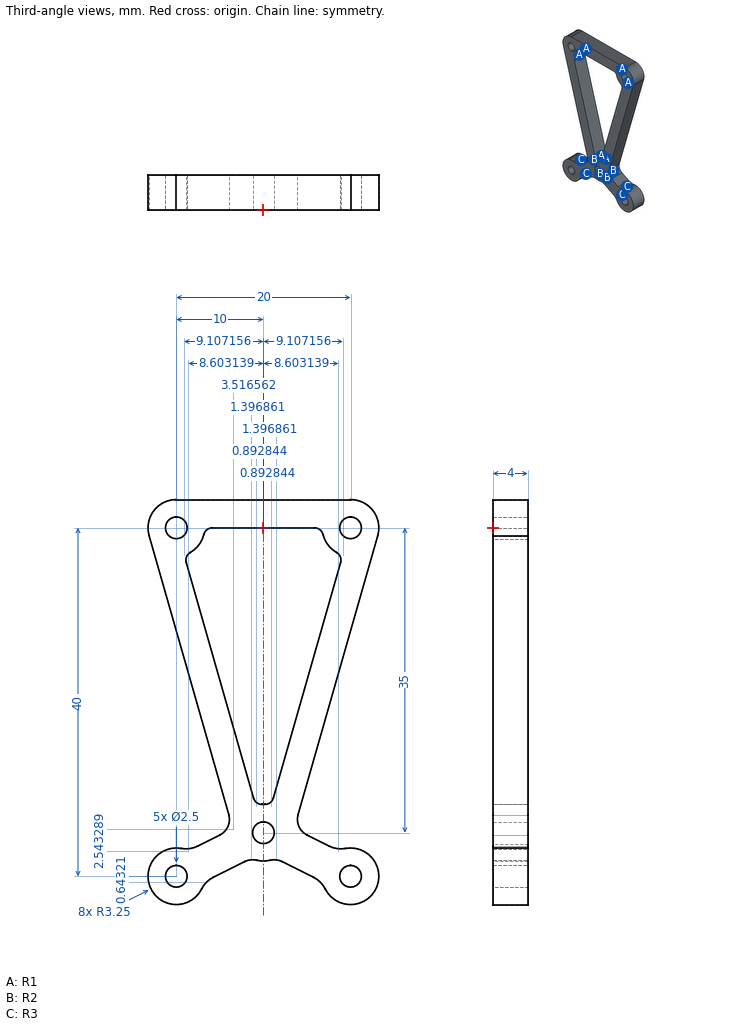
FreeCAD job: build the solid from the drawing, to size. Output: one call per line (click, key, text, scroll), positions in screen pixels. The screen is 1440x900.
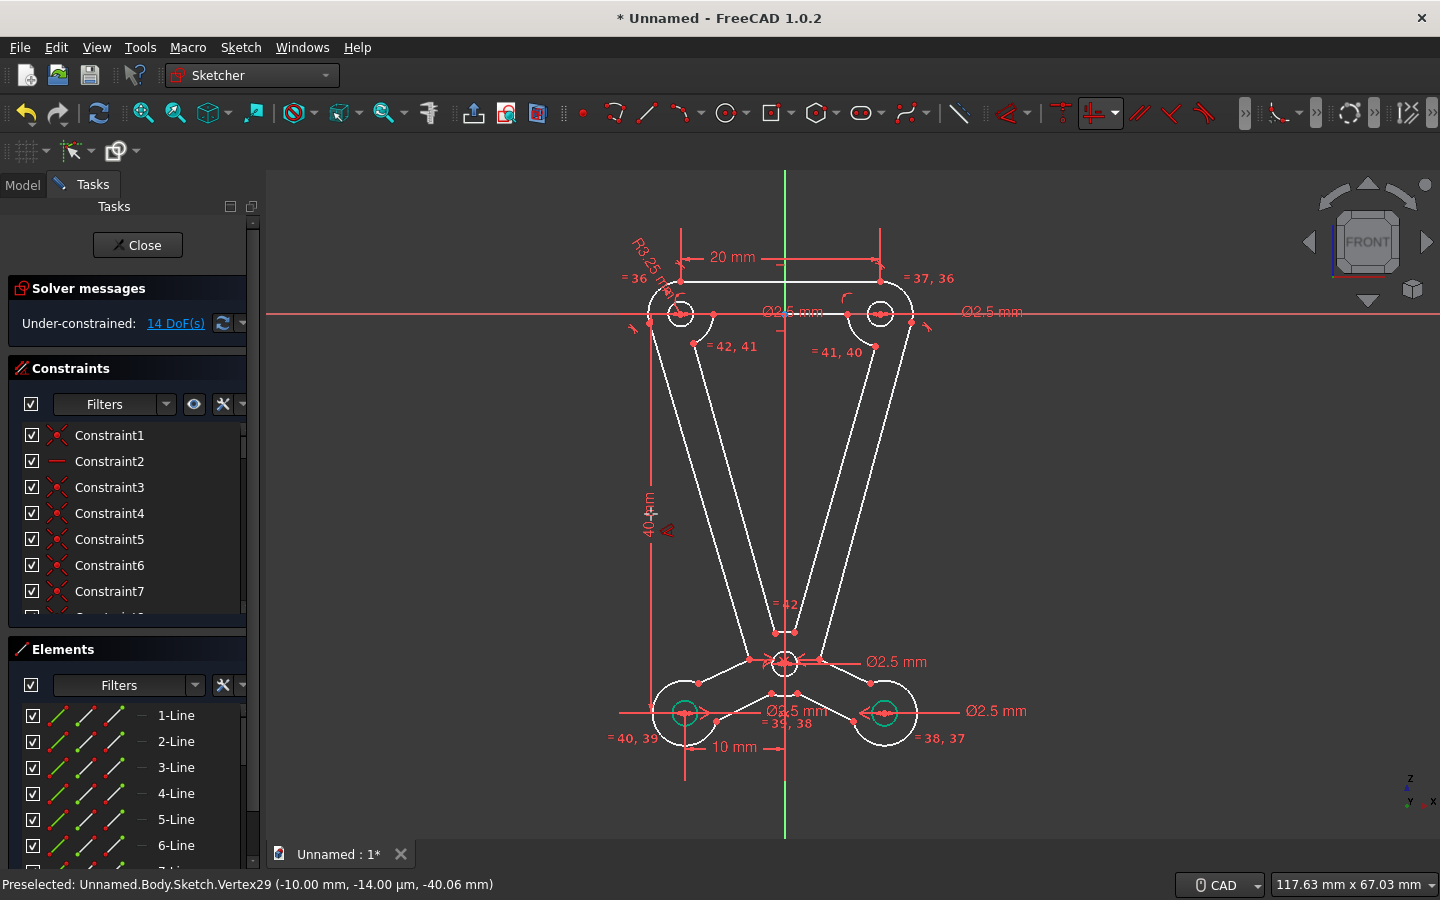
click(785, 664)
click(819, 489)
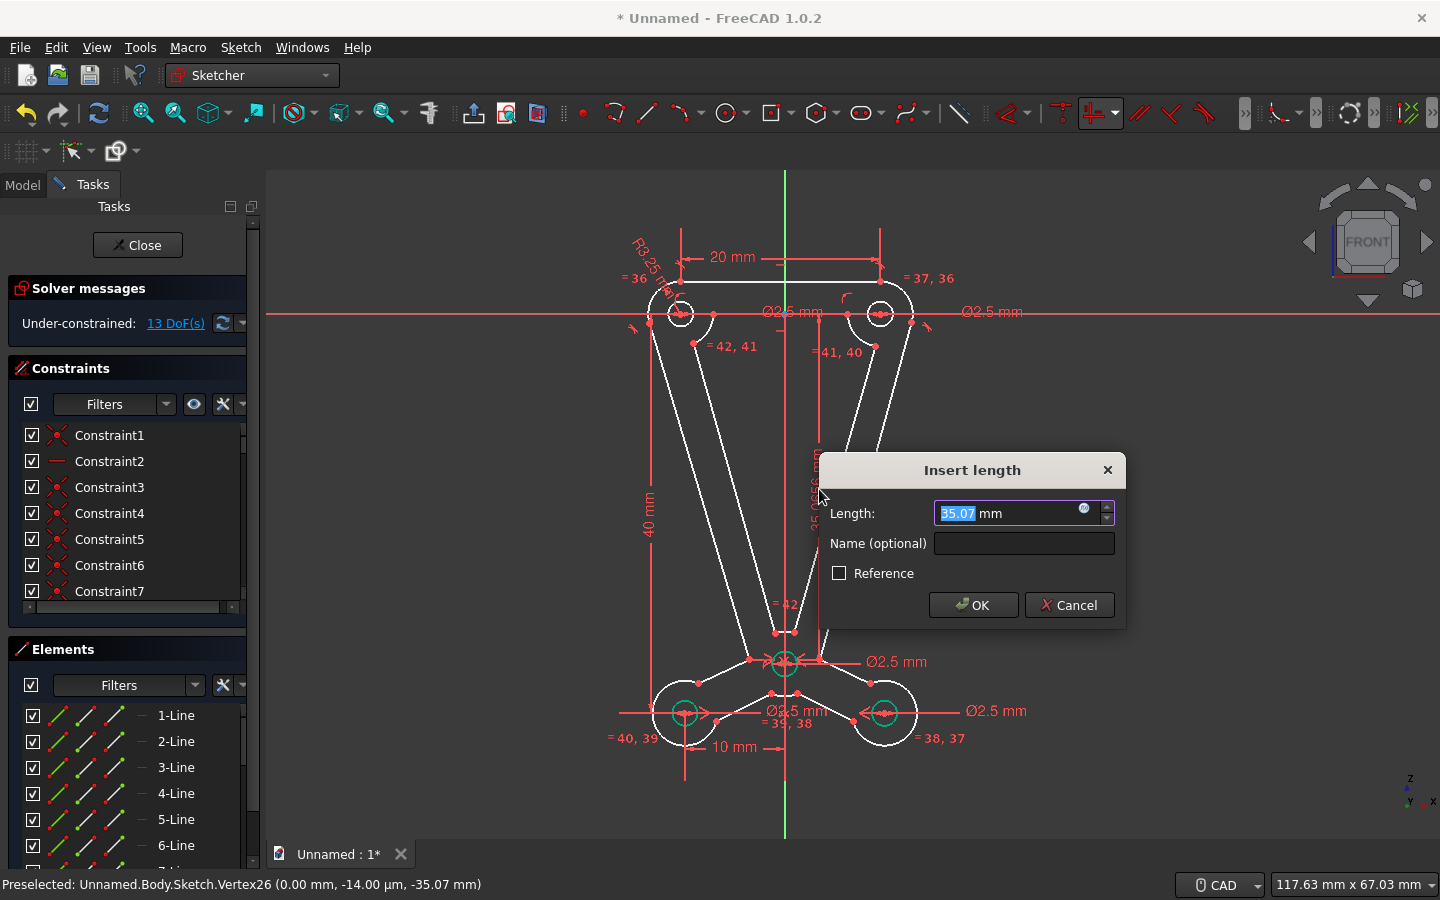
text(35)
key(Return)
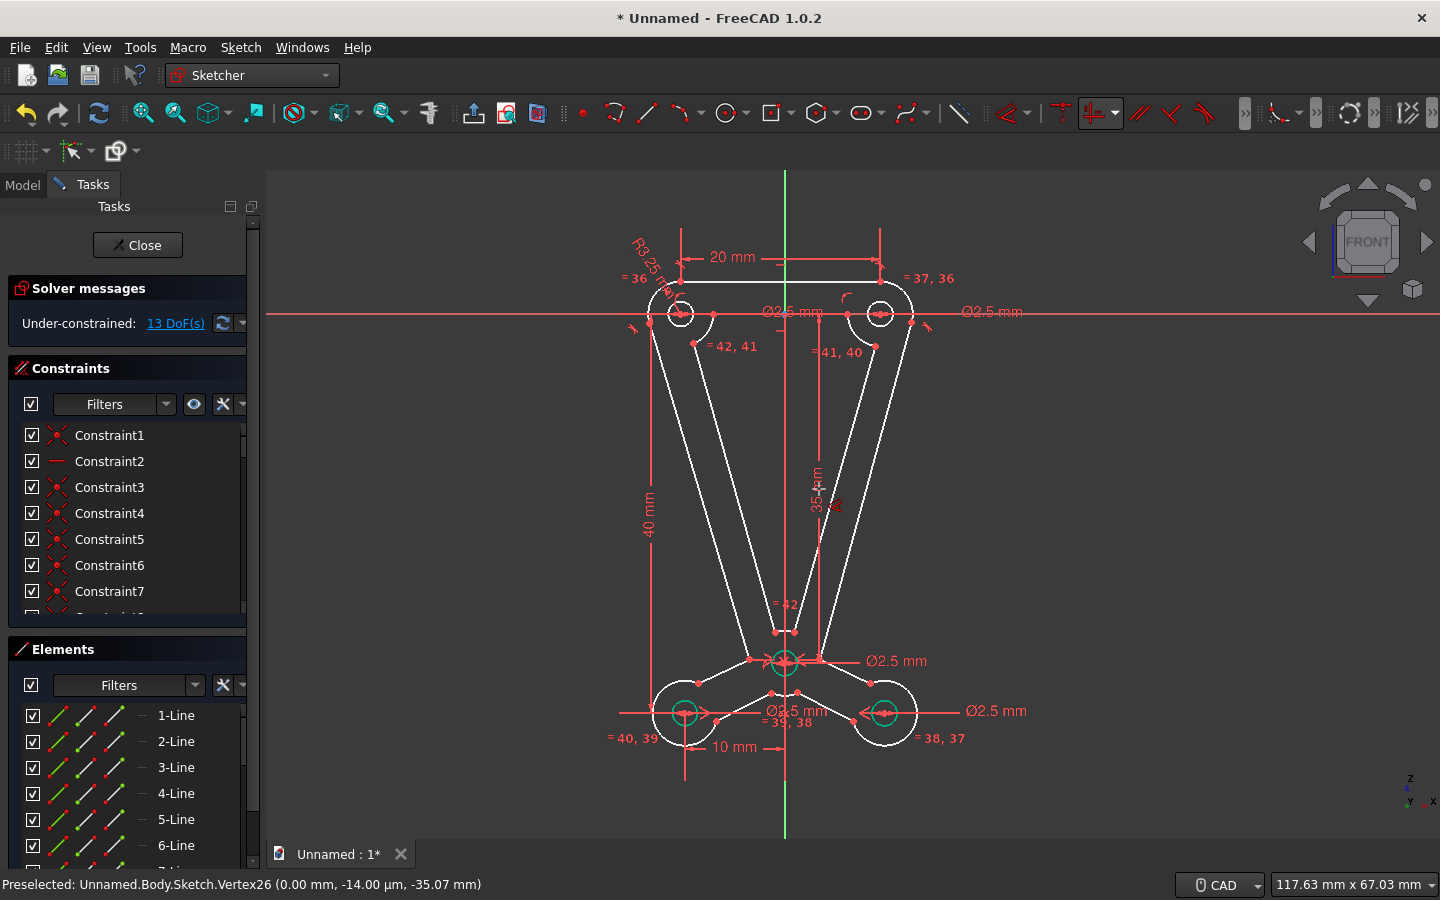
click(681, 314)
click(733, 348)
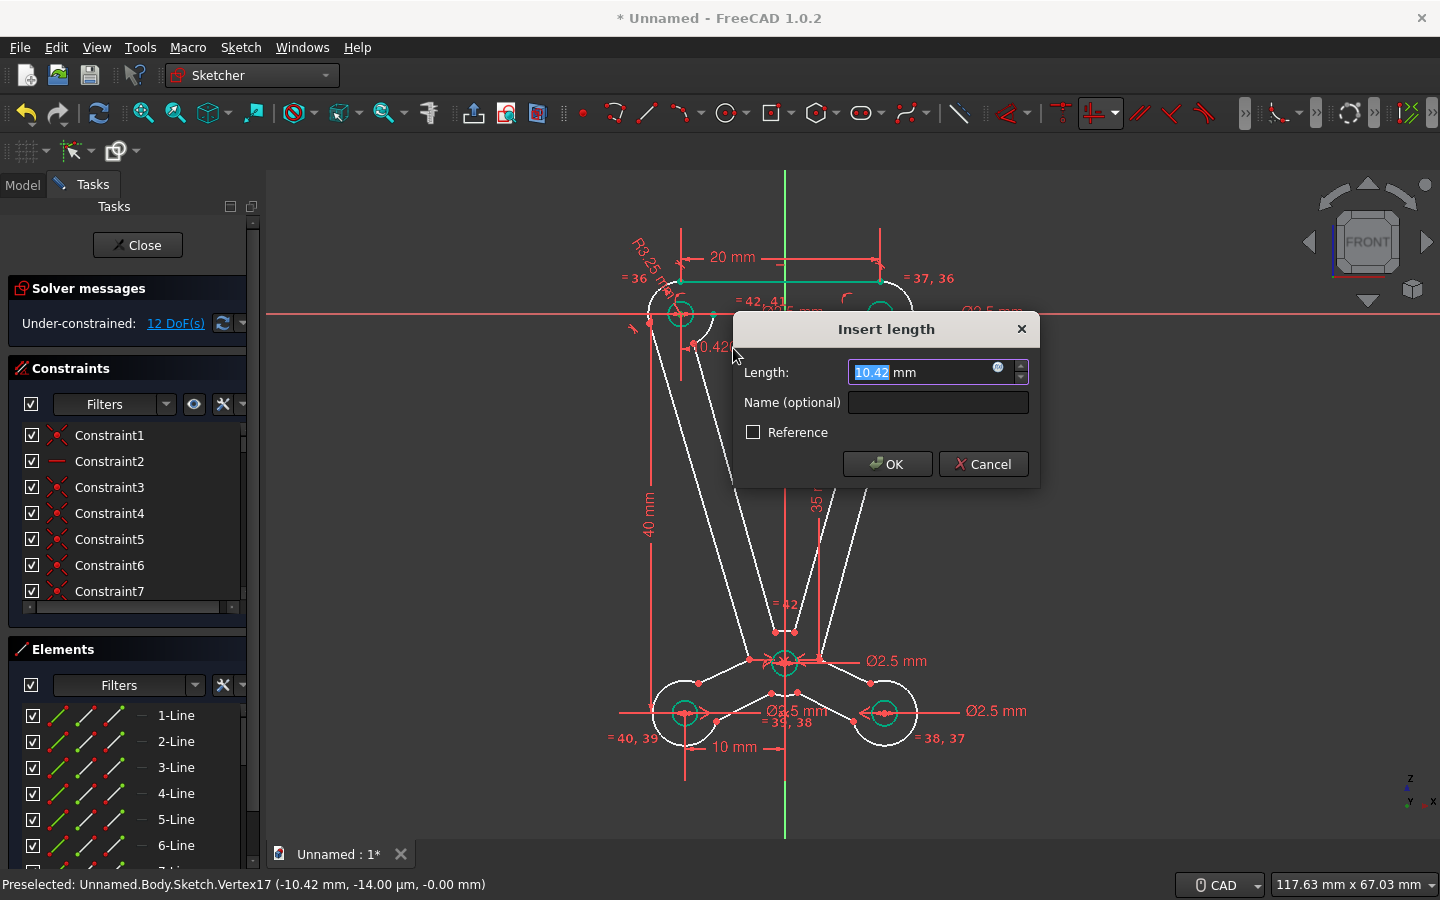
text(10)
key(Return)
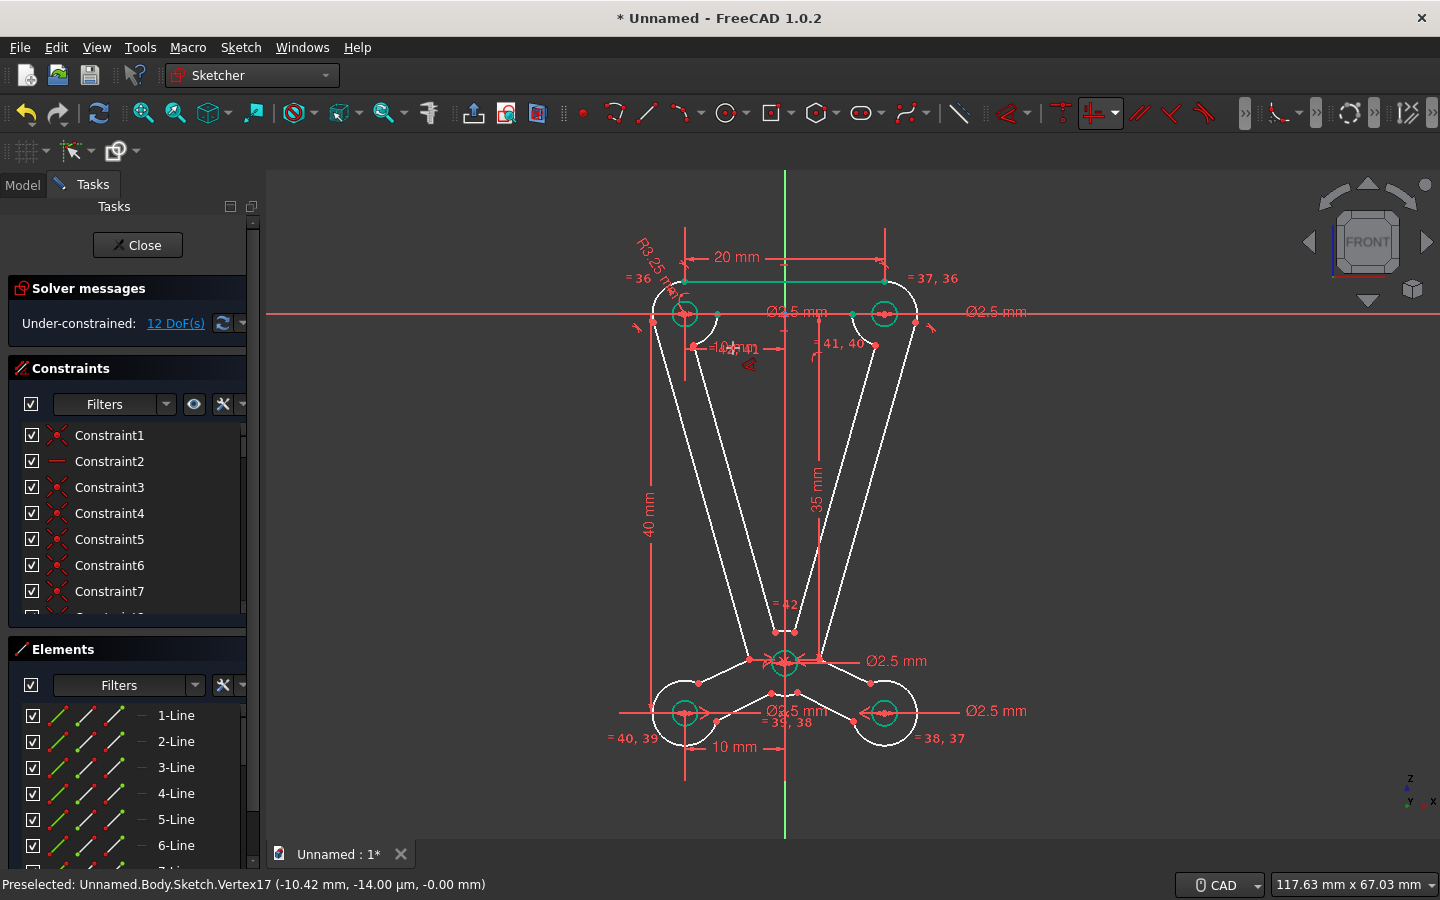
scroll(716, 721, up, 10)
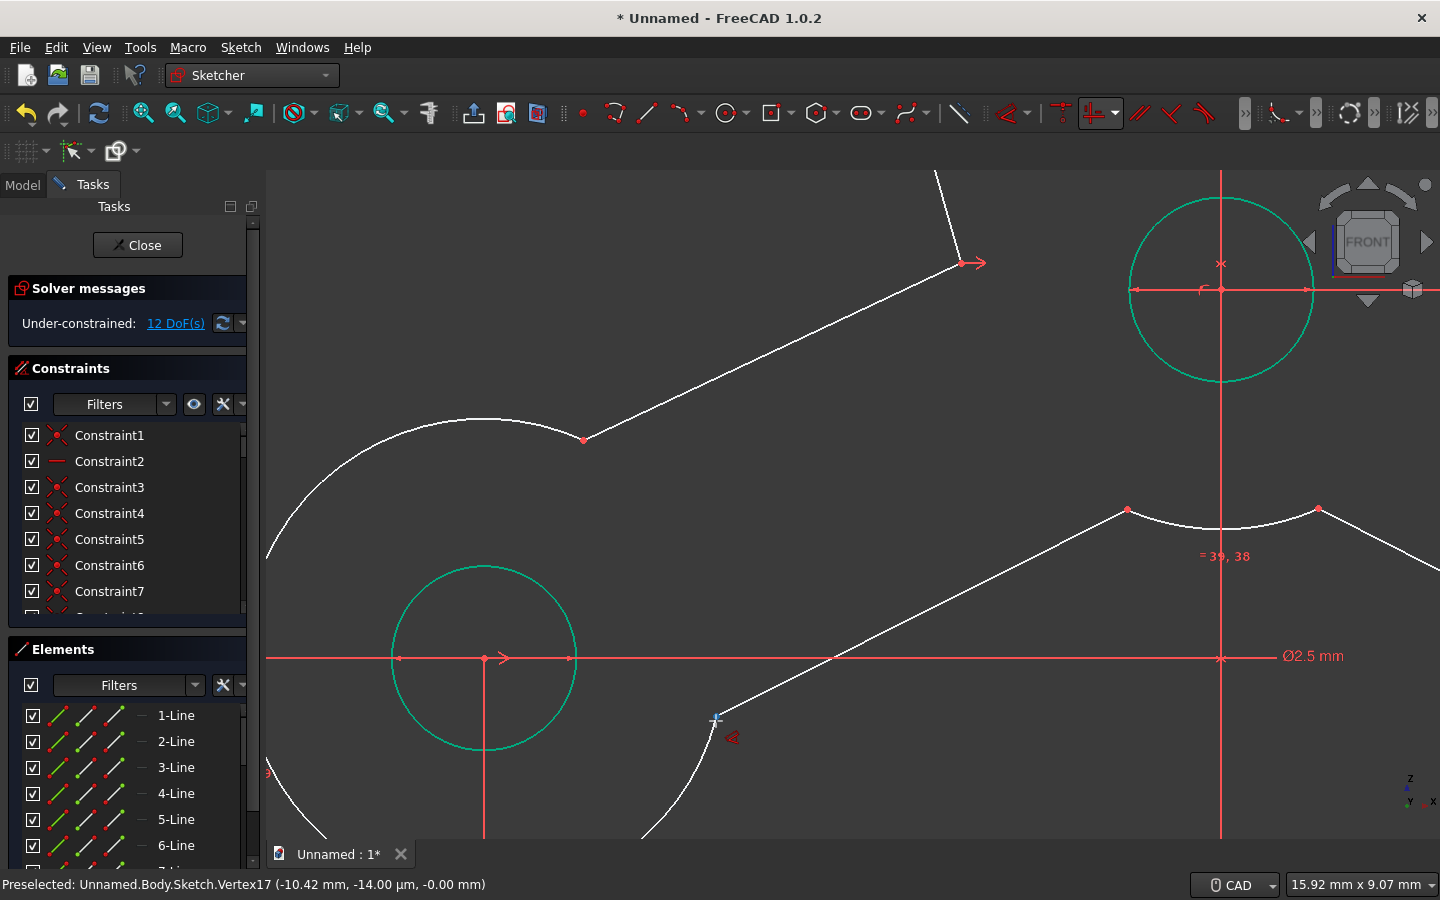
click(717, 716)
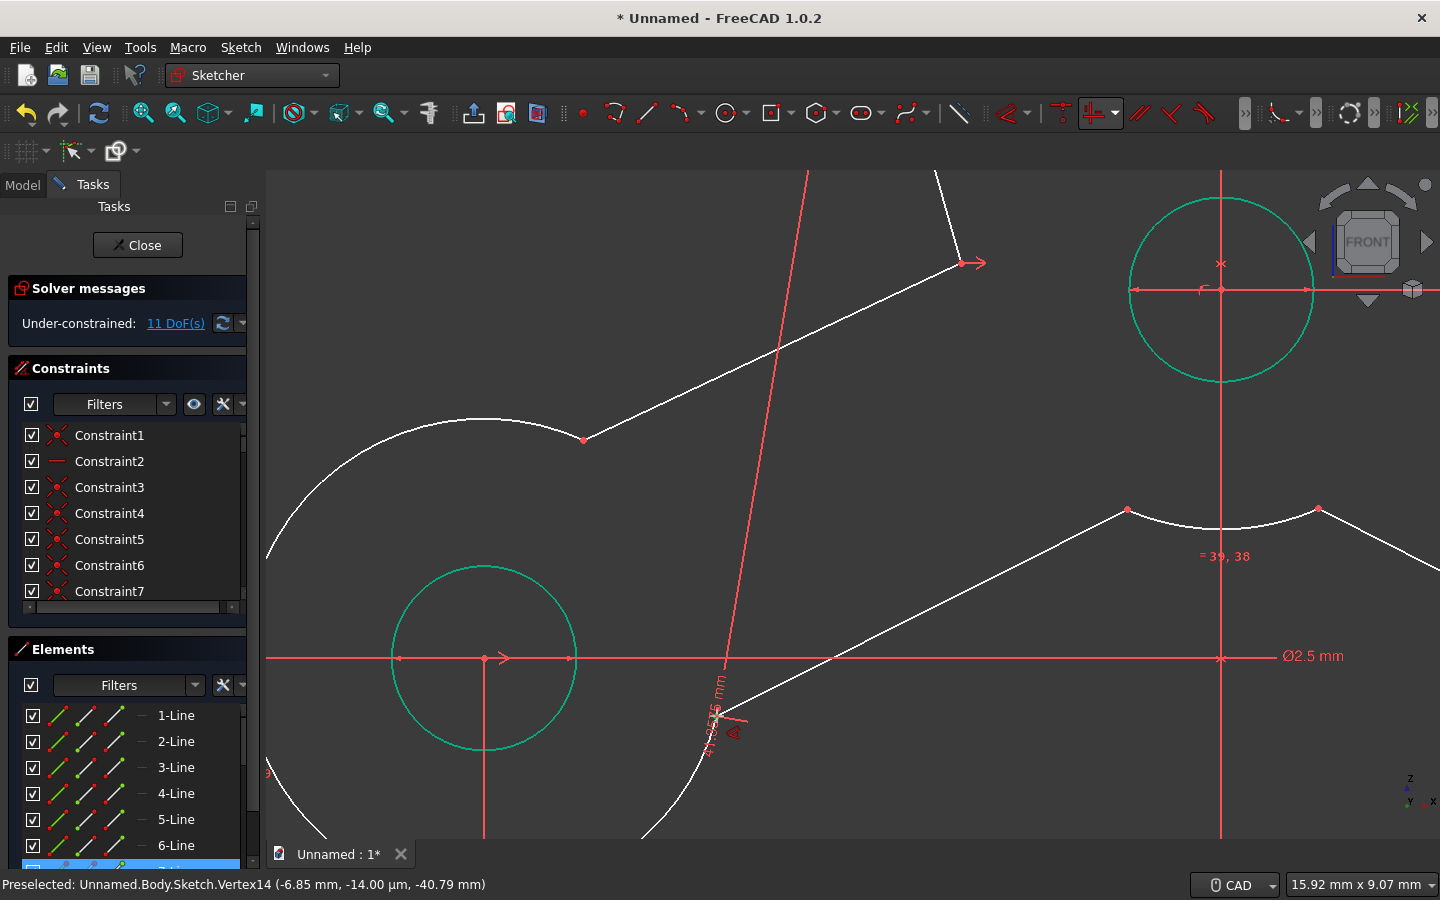
click(484, 658)
click(450, 687)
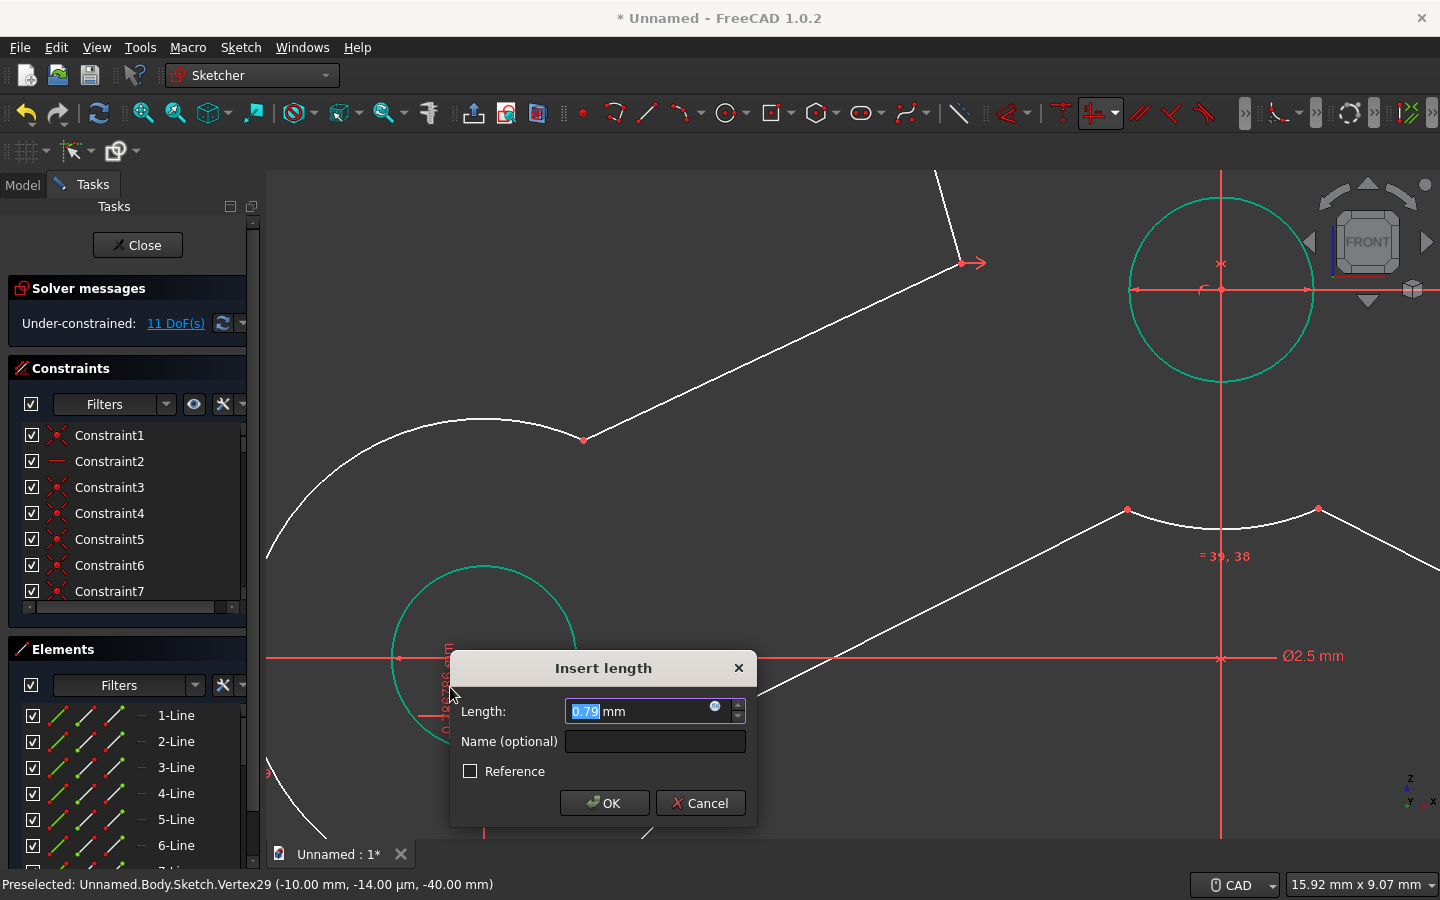
text(0.64321)
key(Return)